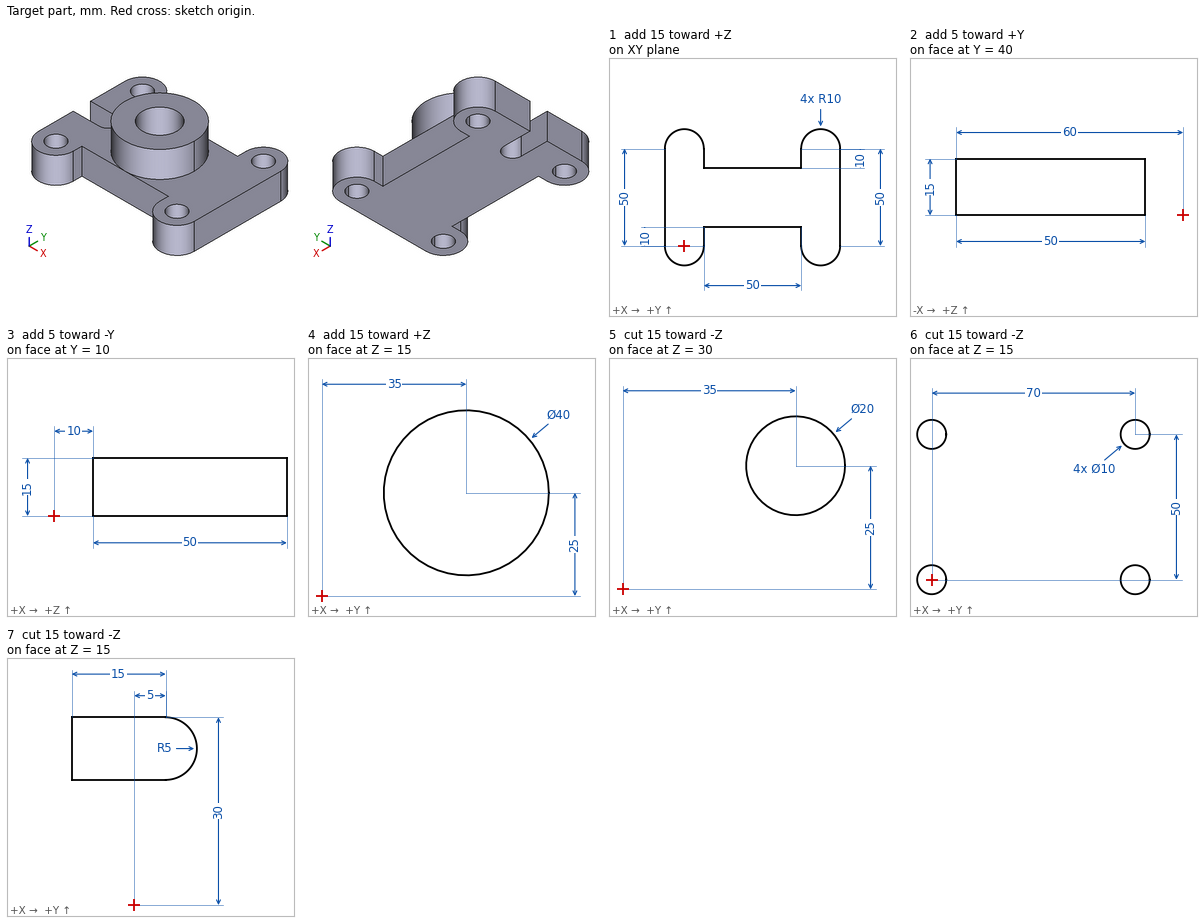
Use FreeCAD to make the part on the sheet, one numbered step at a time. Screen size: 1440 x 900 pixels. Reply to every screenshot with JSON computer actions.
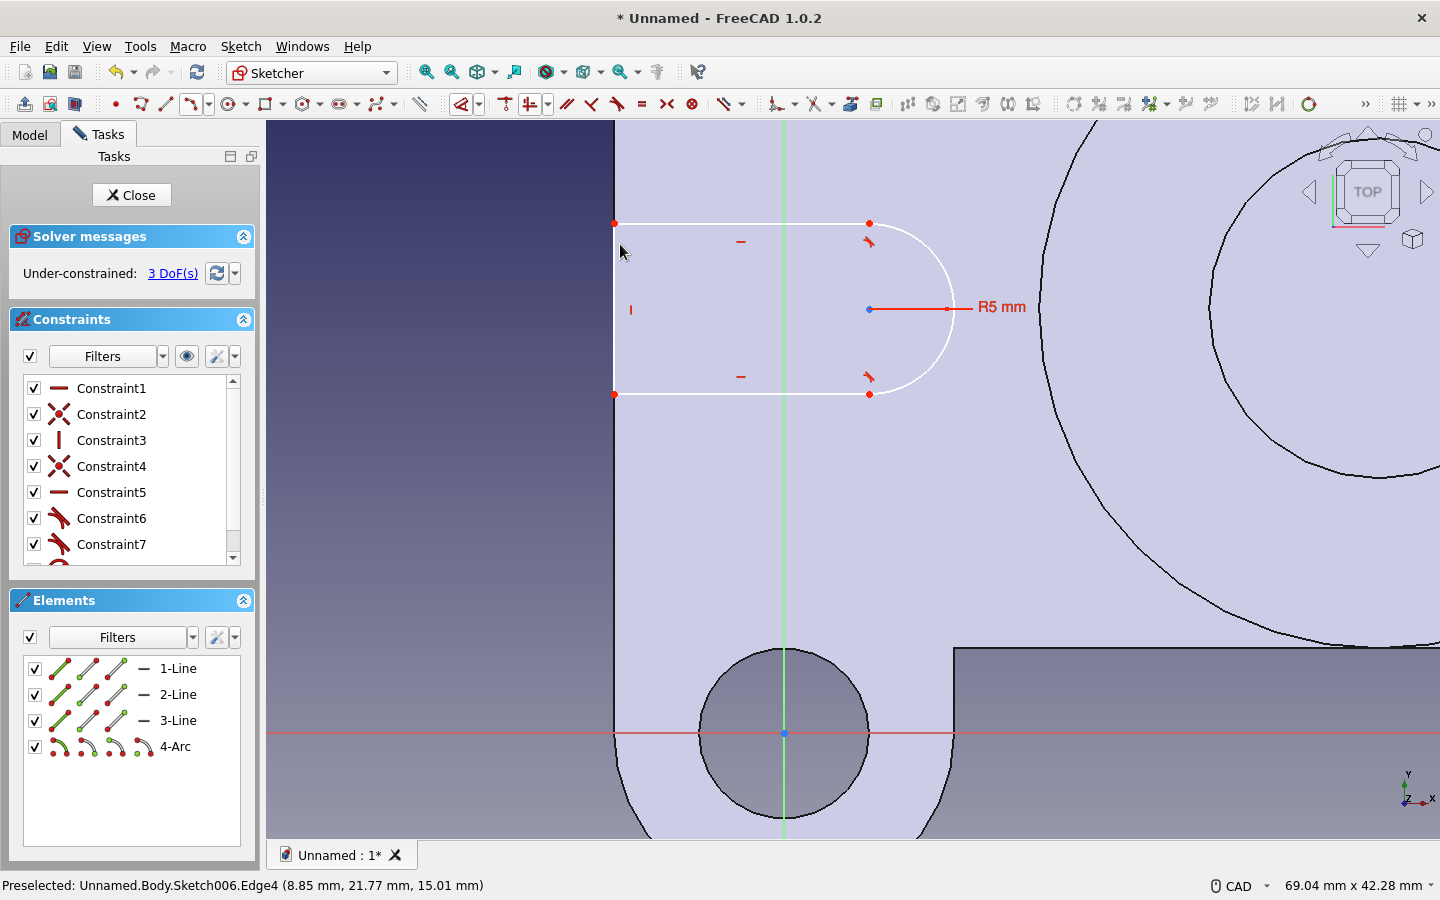
{"action": "left_click", "coordinate": [690, 224]}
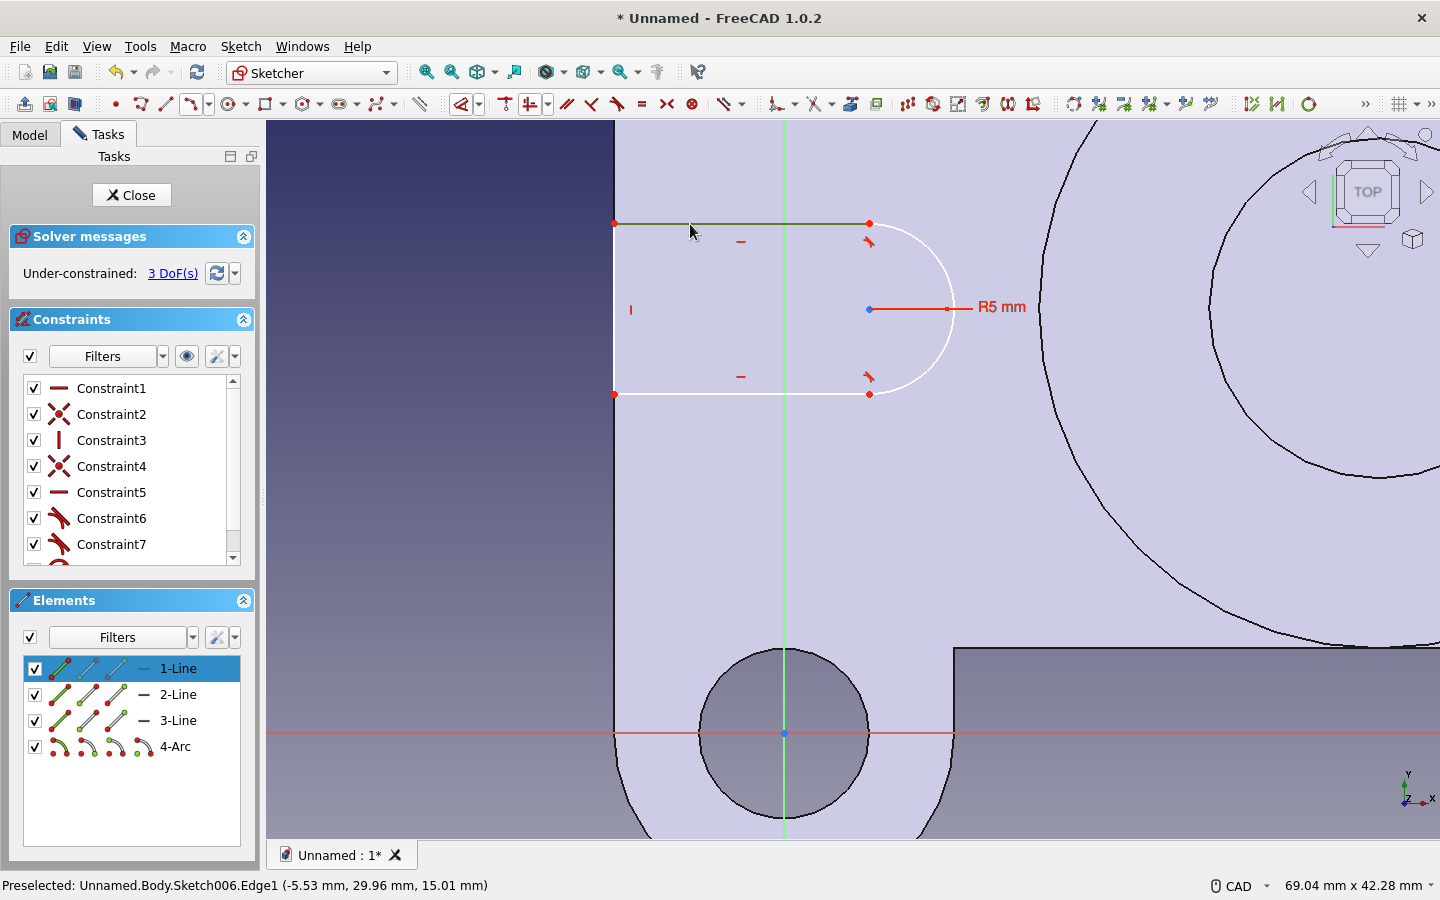
{"action": "key", "text": "l"}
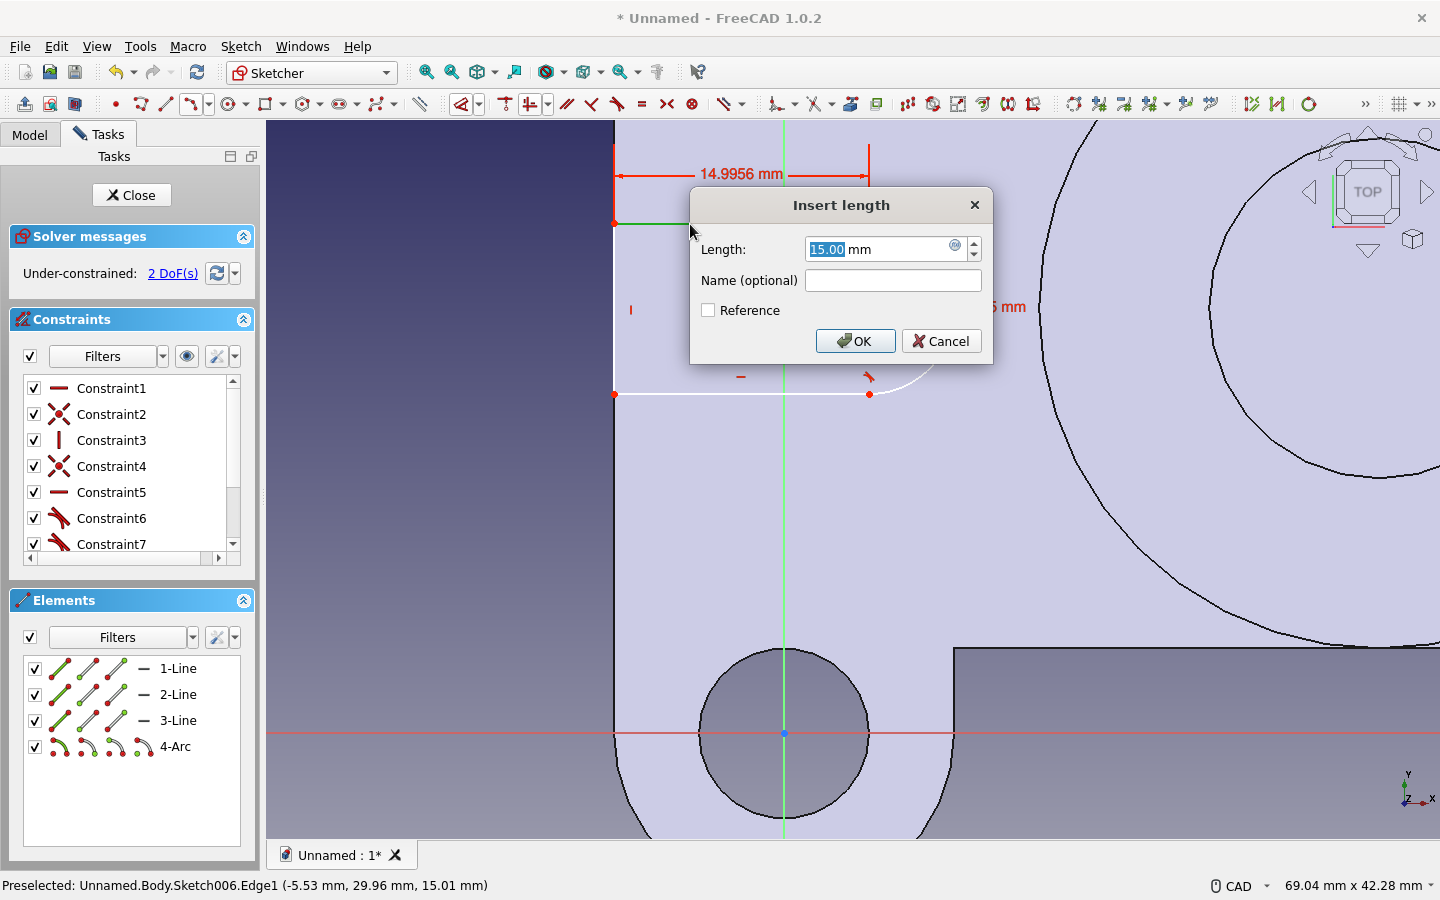
{"action": "type", "text": "15"}
{"action": "key", "text": "Return"}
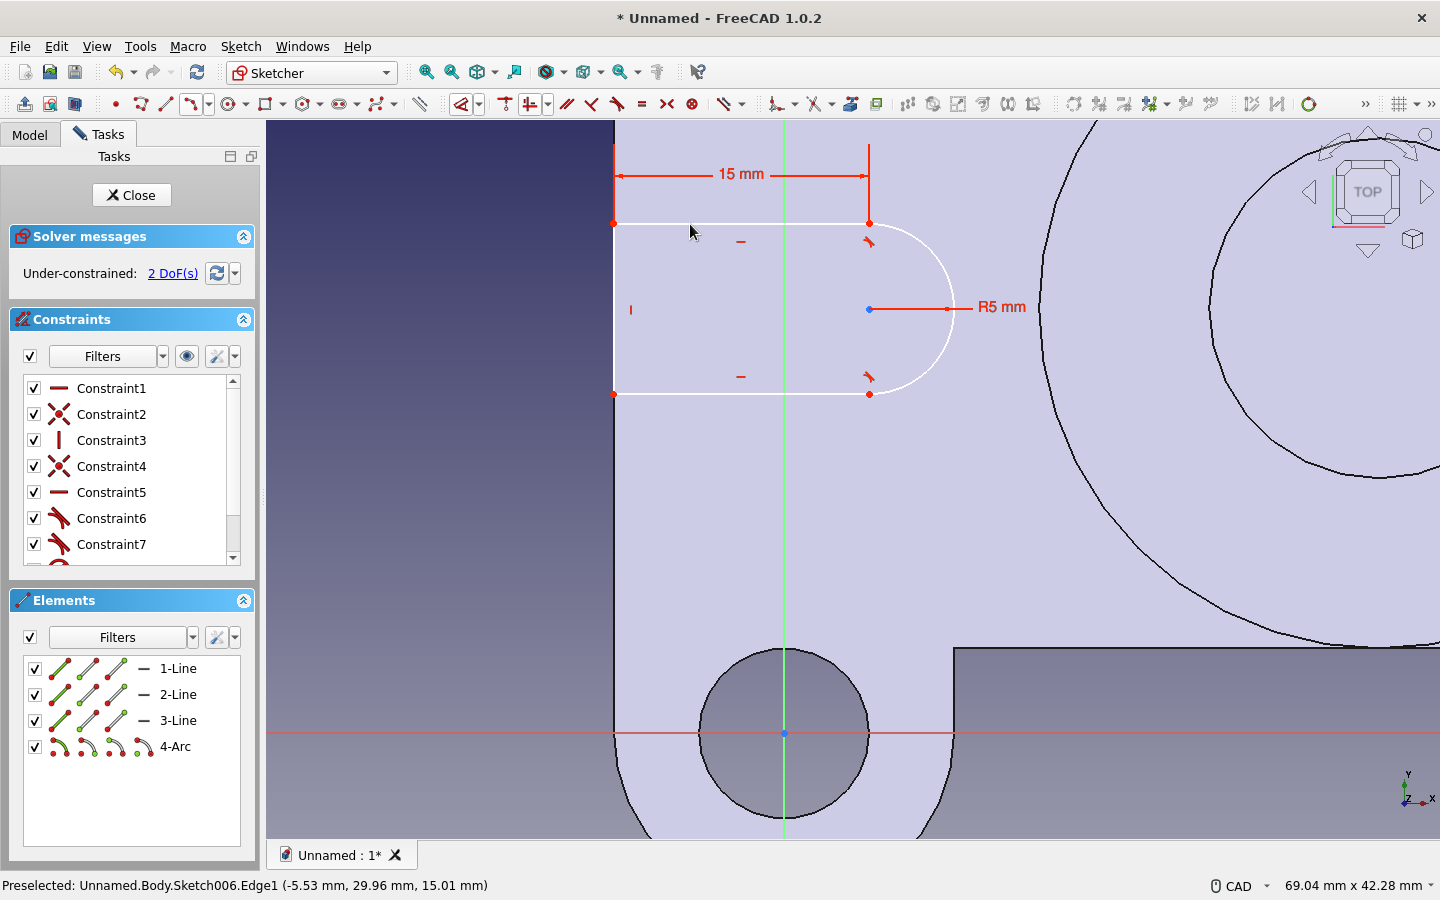
{"action": "left_click", "coordinate": [869, 224]}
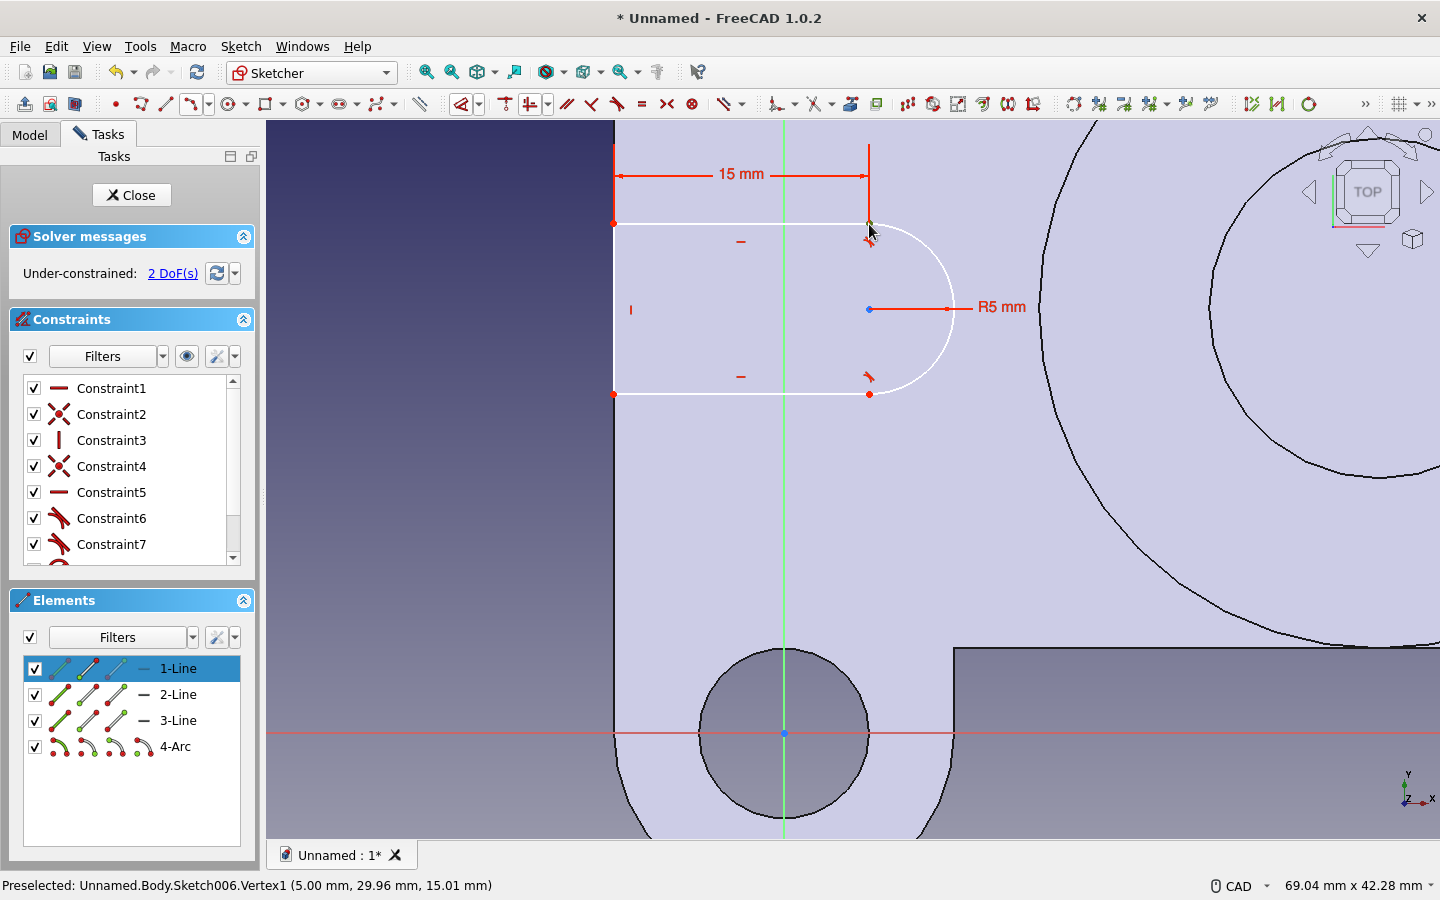
{"action": "left_click", "coordinate": [478, 104]}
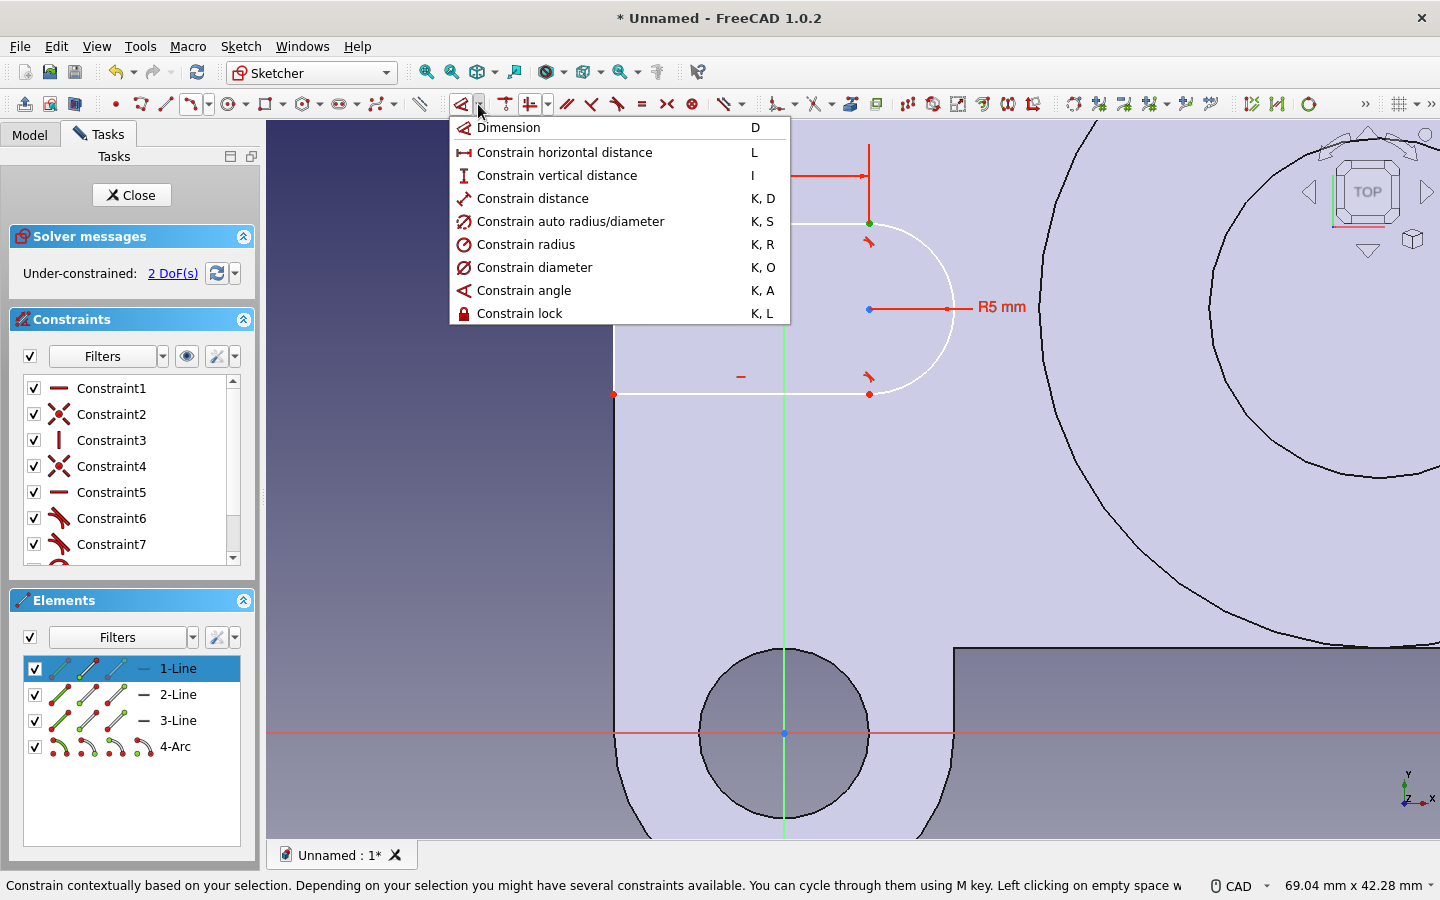
{"action": "left_click", "coordinate": [620, 152]}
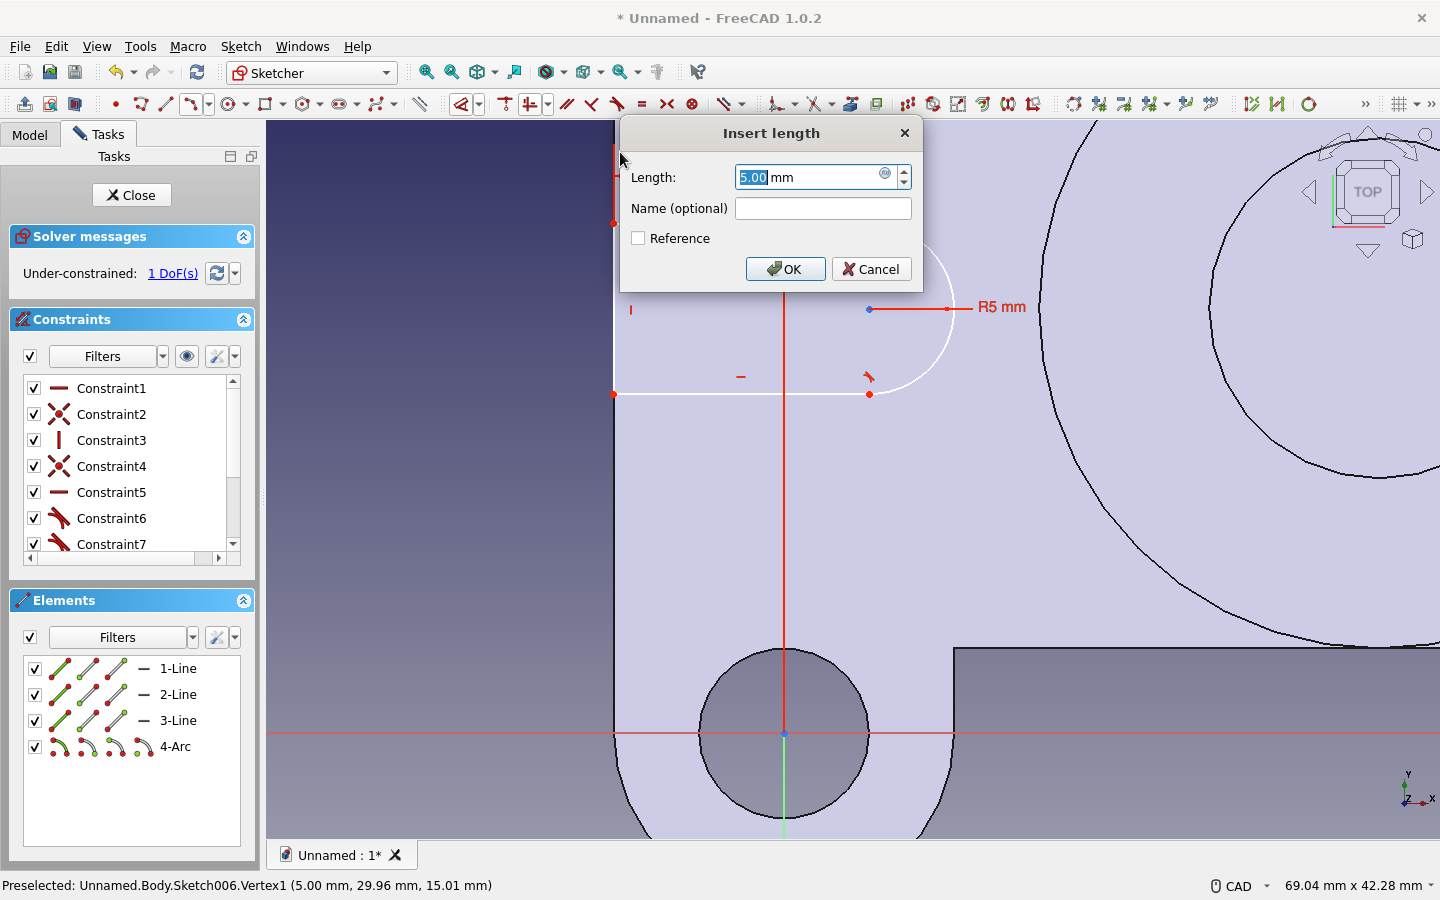
{"action": "type", "text": "5"}
{"action": "key", "text": "Return"}